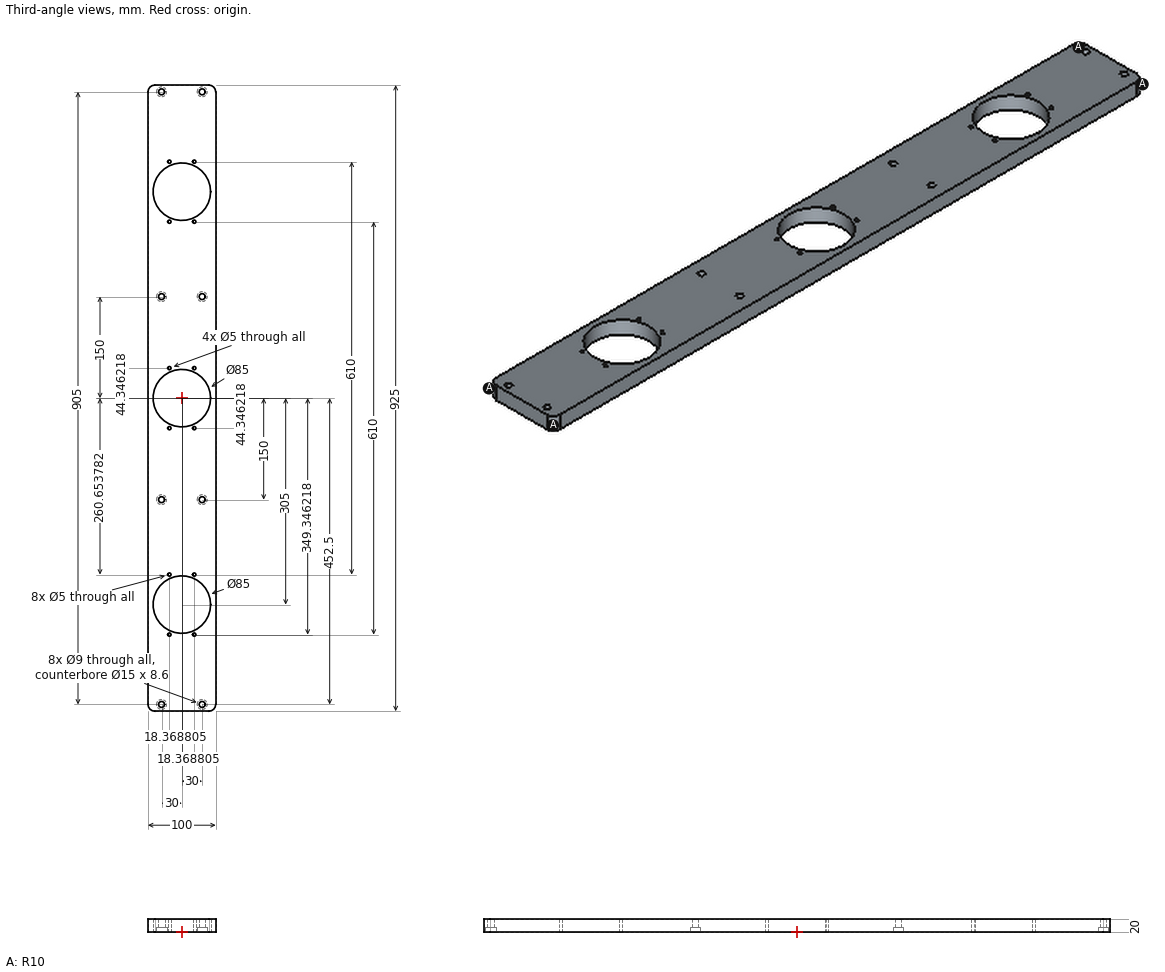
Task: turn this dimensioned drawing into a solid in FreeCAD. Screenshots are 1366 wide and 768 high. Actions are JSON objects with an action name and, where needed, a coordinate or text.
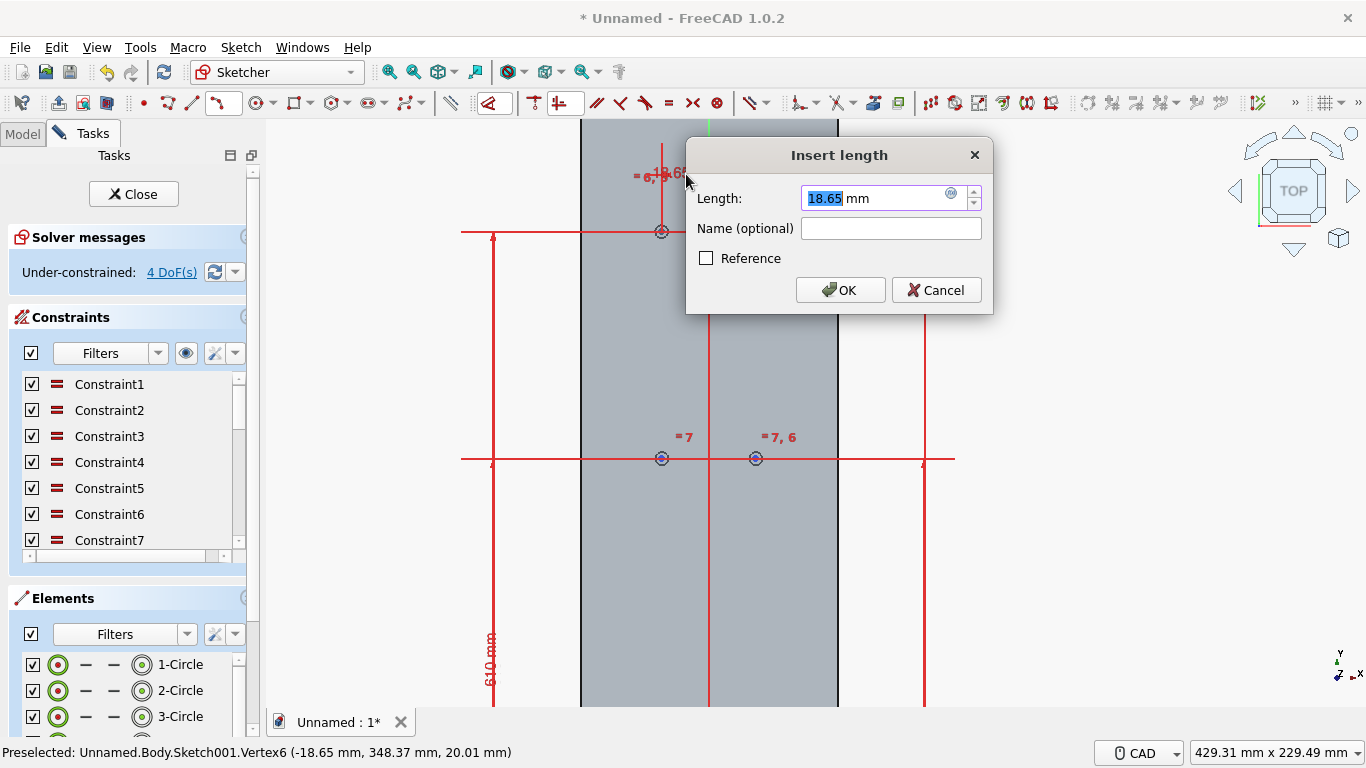
{"action": "type", "text": "18.368805"}
{"action": "key", "text": "Return"}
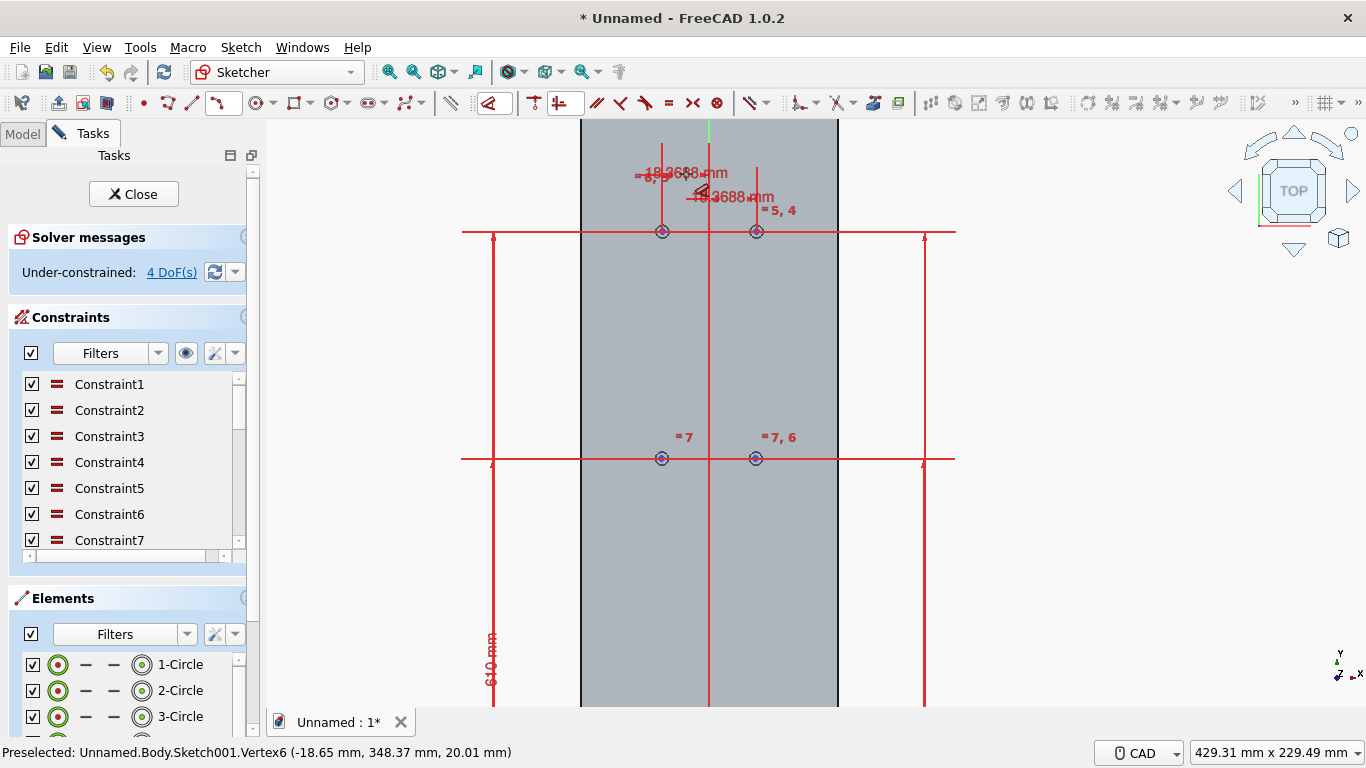
{"action": "left_click", "coordinate": [756, 459]}
{"action": "left_click", "coordinate": [733, 425]}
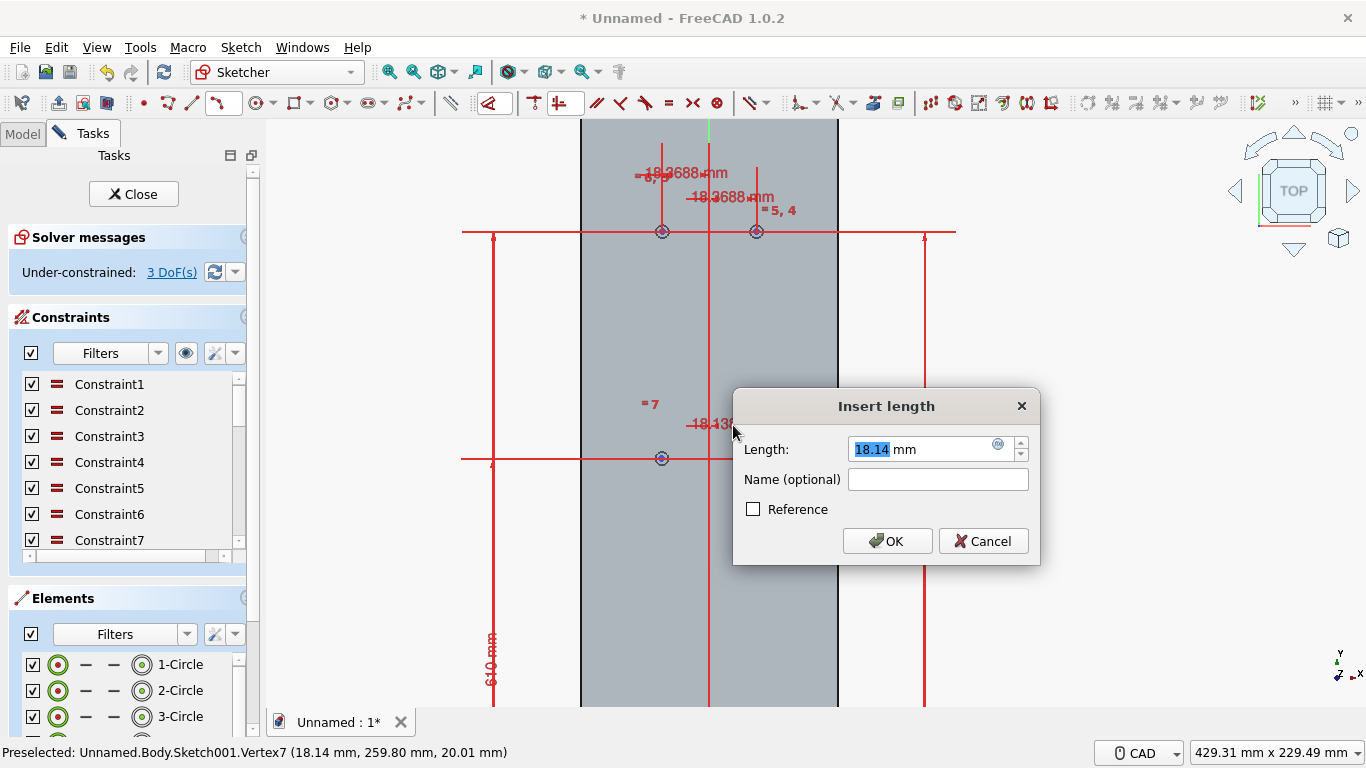
{"action": "type", "text": "18.368805"}
{"action": "key", "text": "Return"}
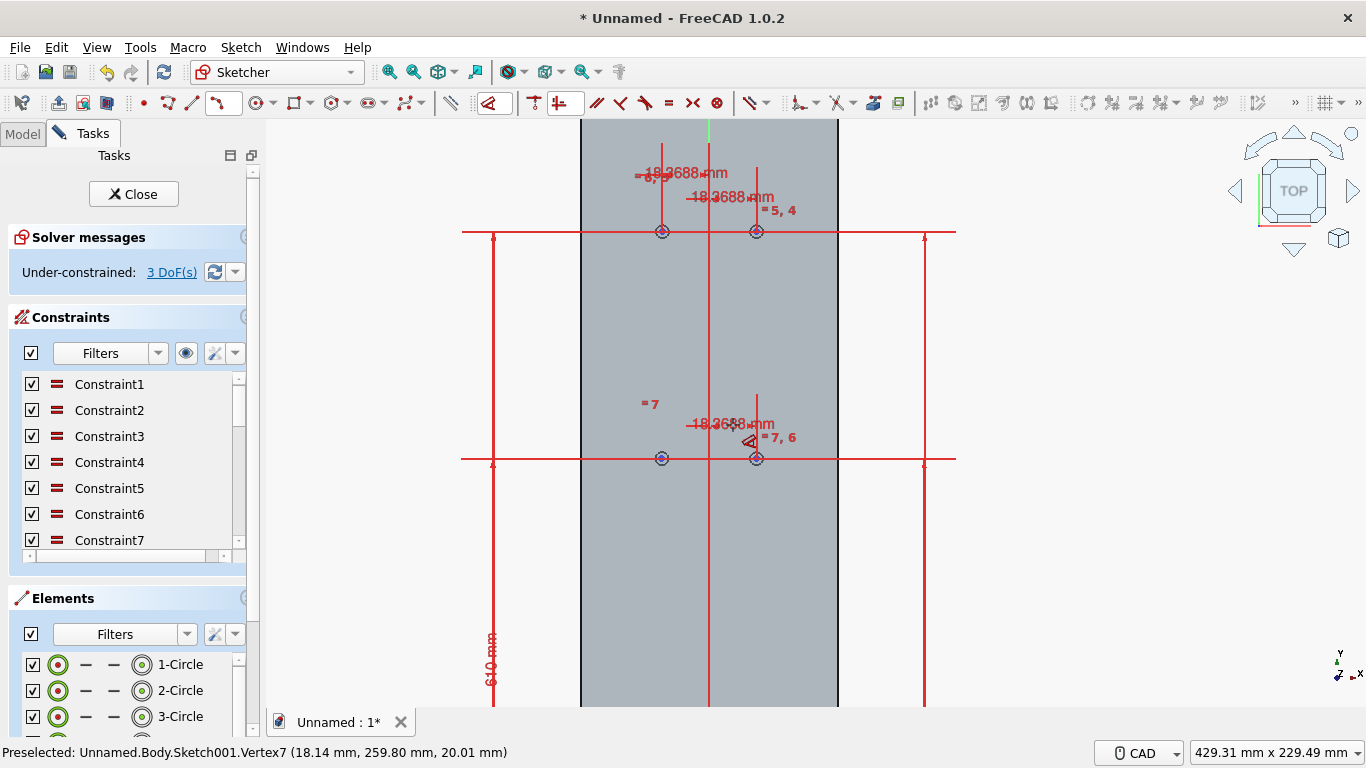
{"action": "left_click", "coordinate": [662, 459]}
{"action": "left_click", "coordinate": [686, 401]}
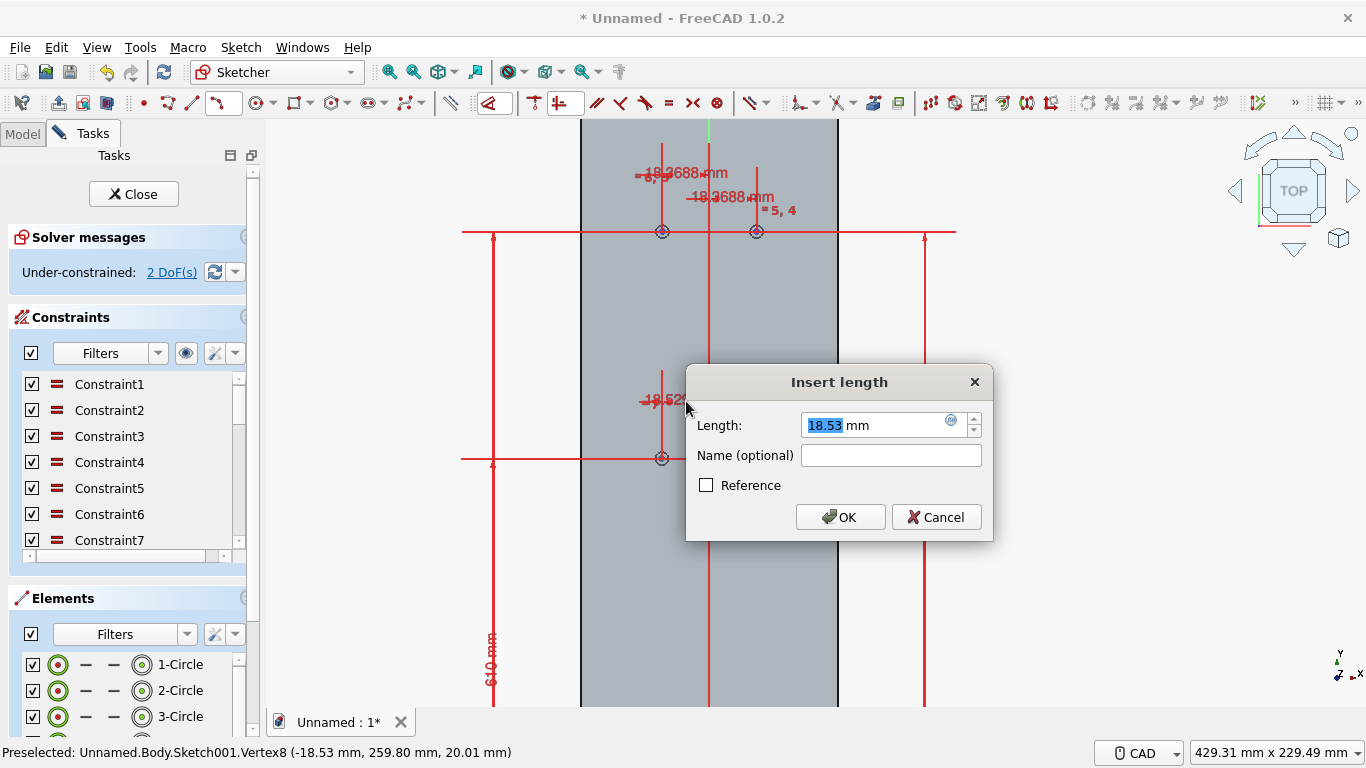
{"action": "type", "text": "18.368805"}
{"action": "key", "text": "Return"}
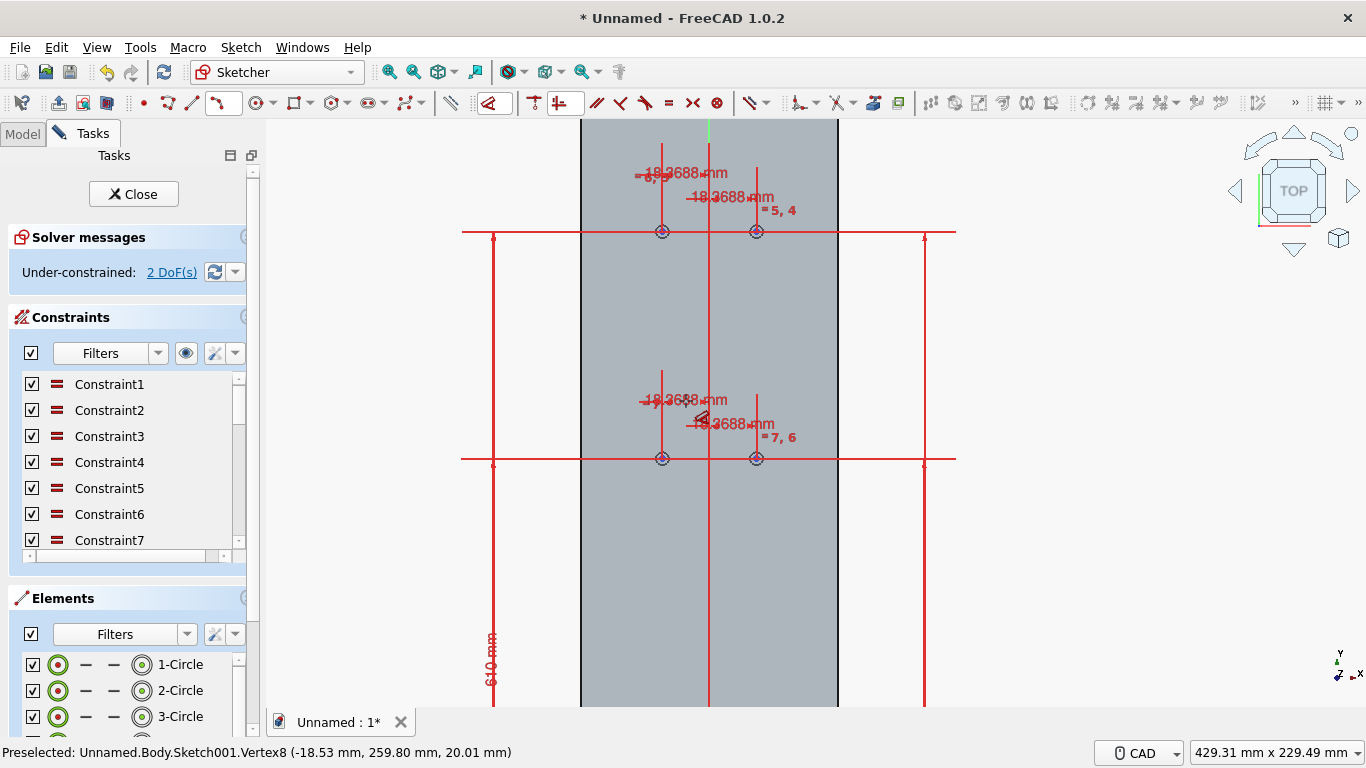
{"action": "scroll", "coordinate": [757, 233], "scroll_direction": "down", "scroll_amount": 8}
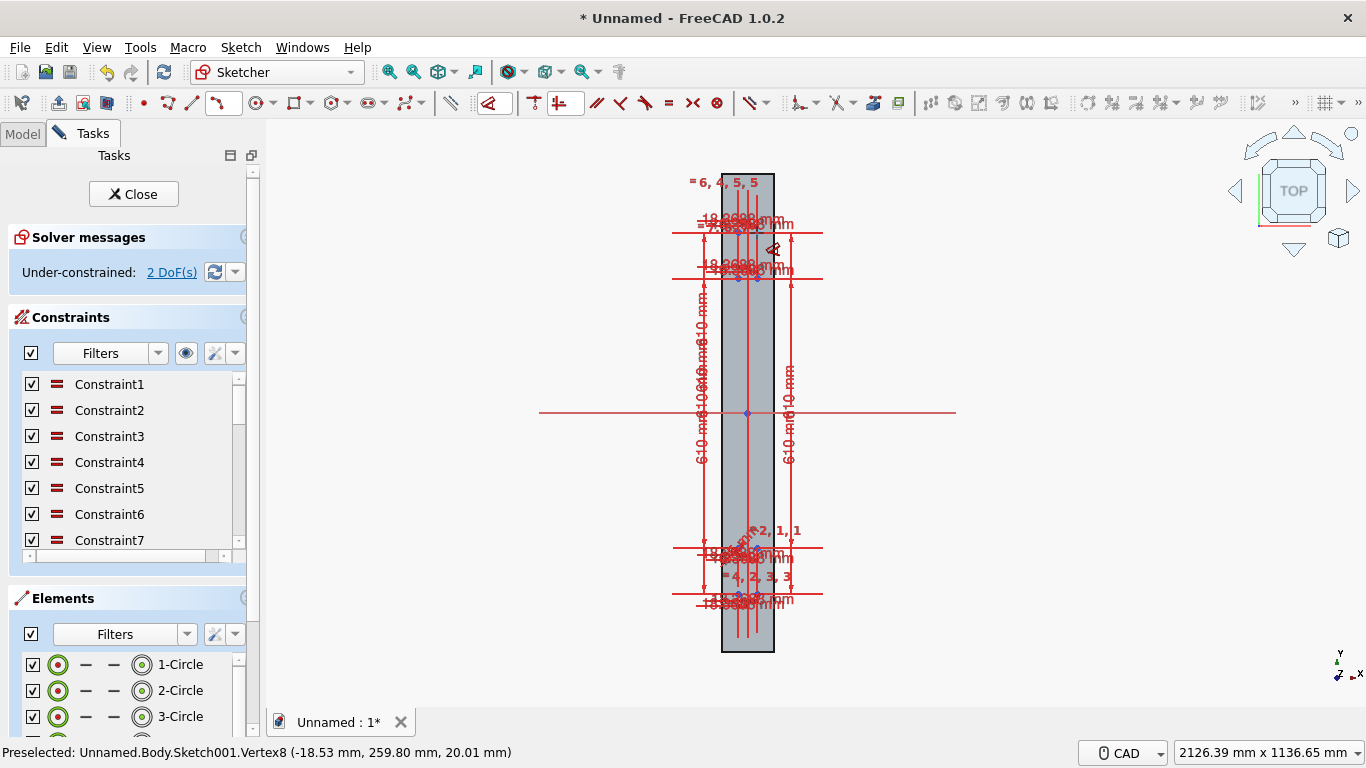
{"action": "left_click", "coordinate": [738, 548]}
{"action": "left_click", "coordinate": [704, 481]}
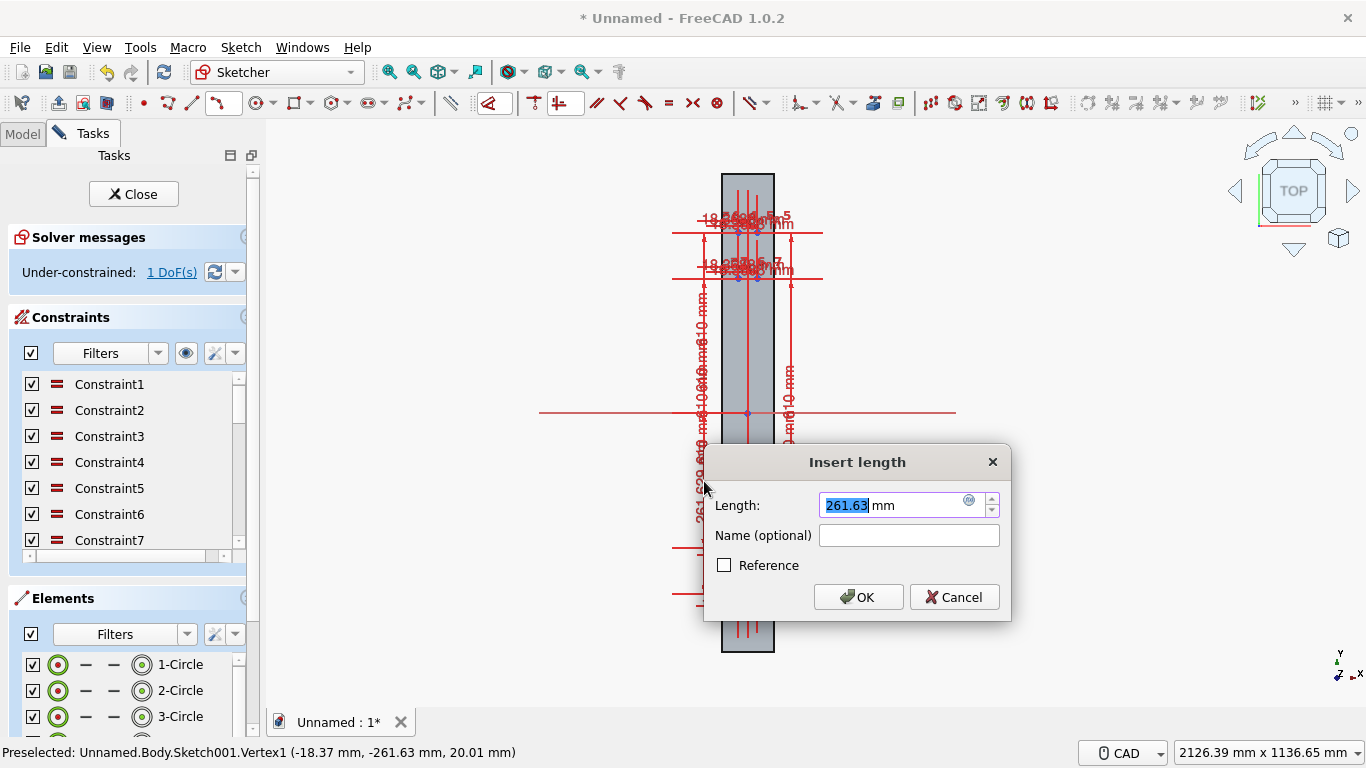
{"action": "type", "text": "260.653782"}
{"action": "key", "text": "Return"}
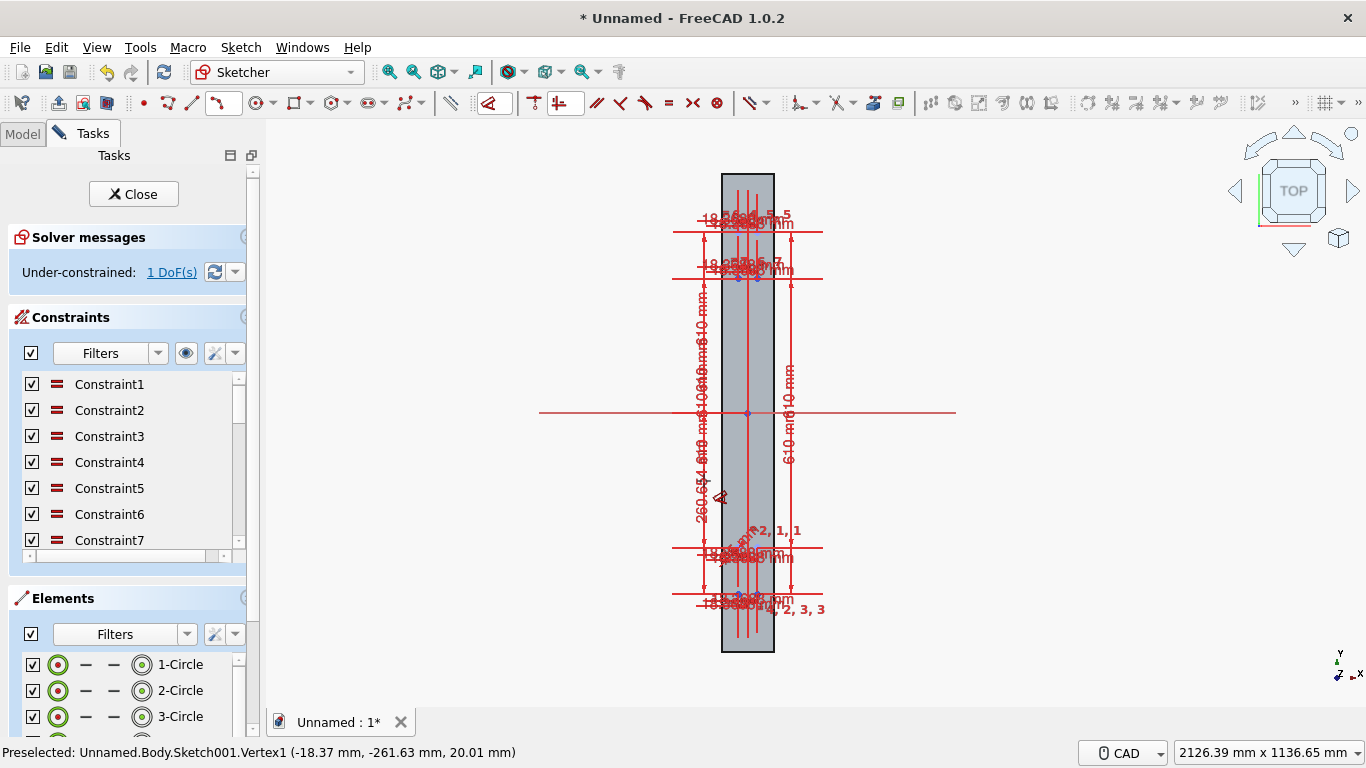
{"action": "left_click", "coordinate": [757, 594]}
{"action": "left_click", "coordinate": [791, 504]}